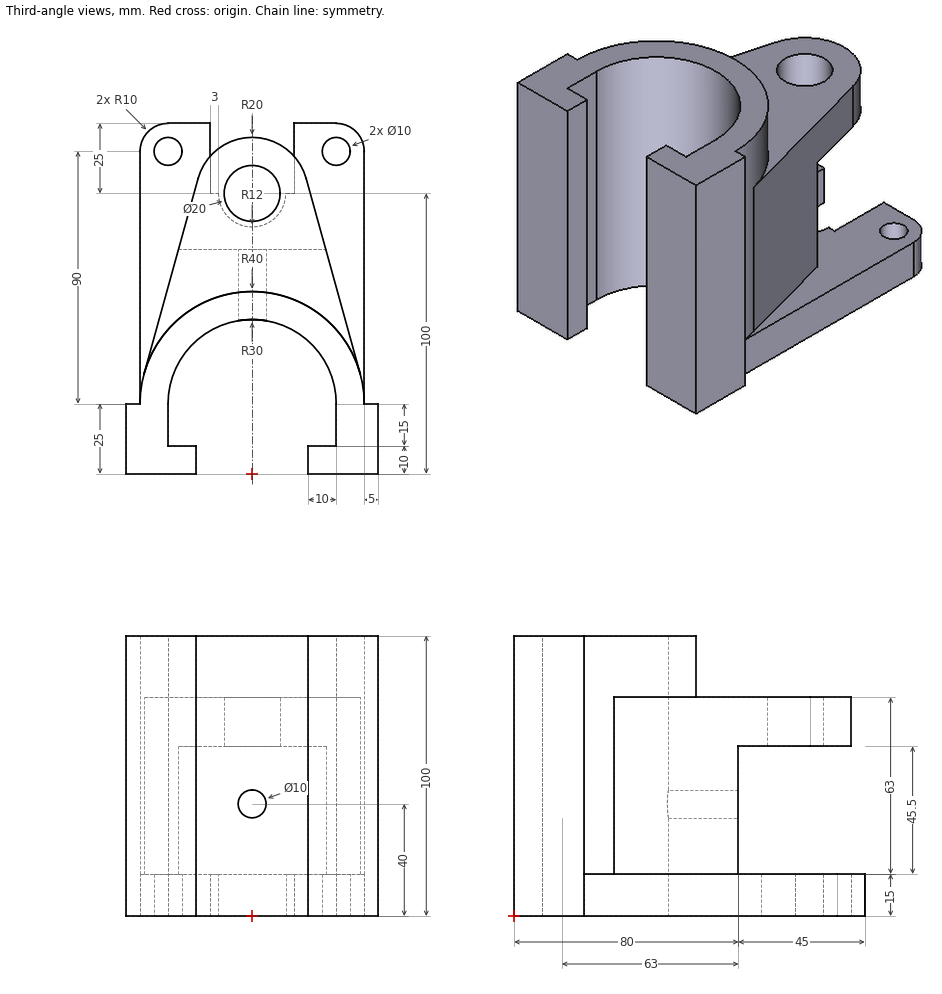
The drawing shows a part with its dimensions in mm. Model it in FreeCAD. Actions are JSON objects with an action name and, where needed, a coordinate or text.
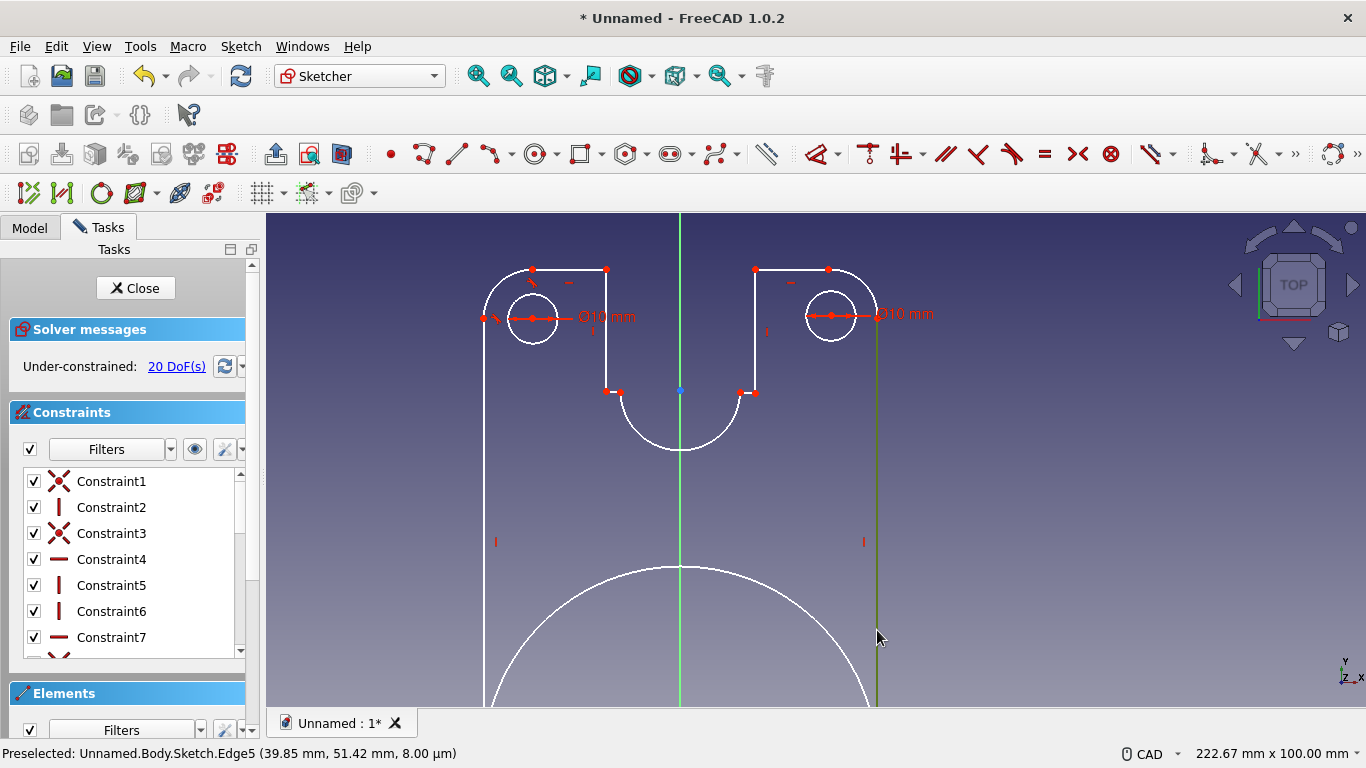
{"action": "left_click", "coordinate": [873, 296]}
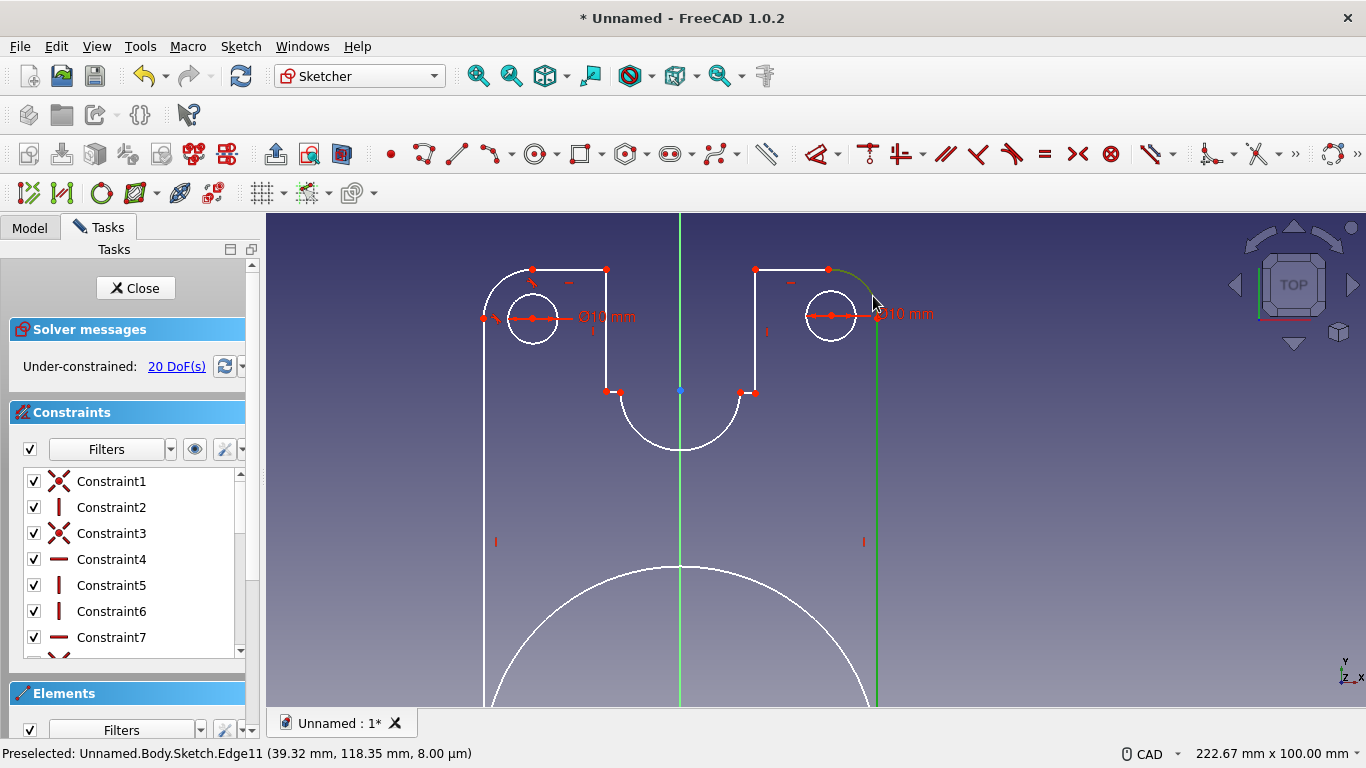
{"action": "key", "text": "t"}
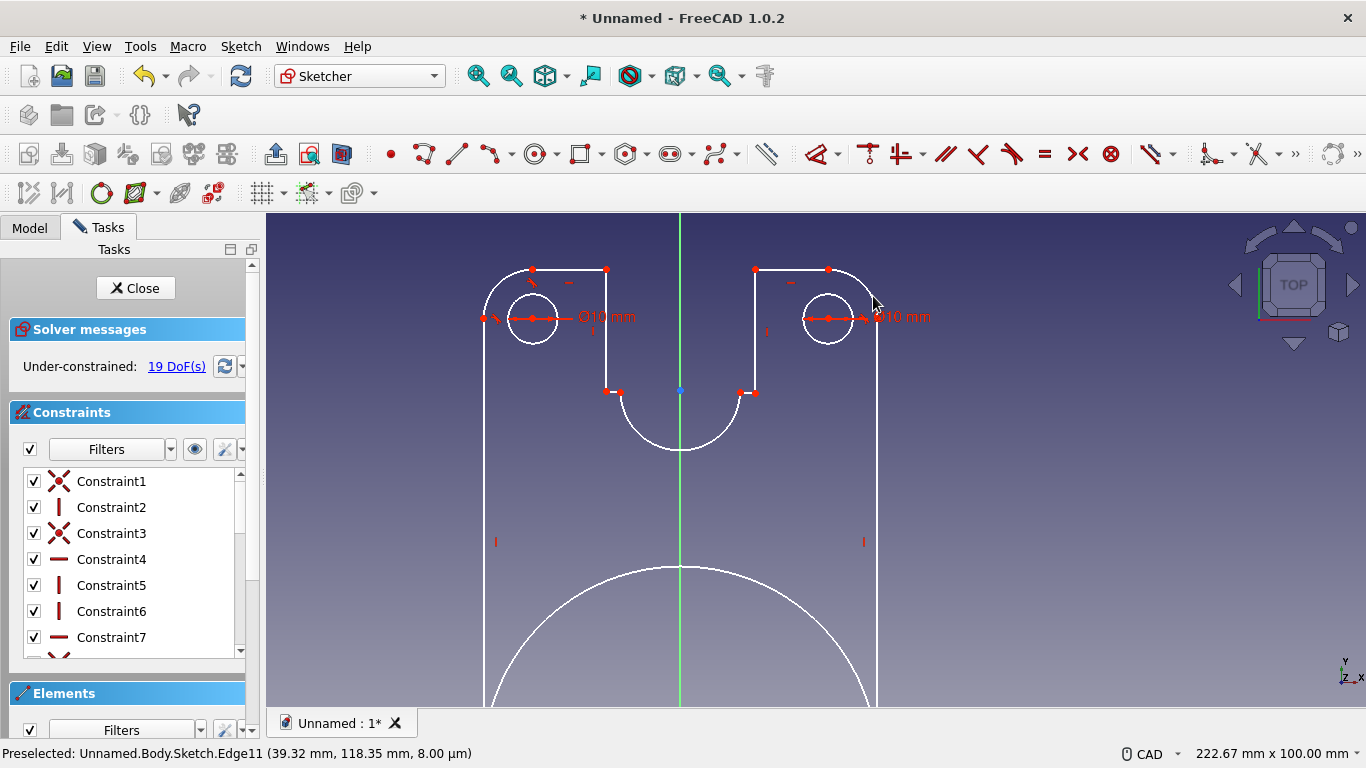
{"action": "left_click", "coordinate": [806, 270]}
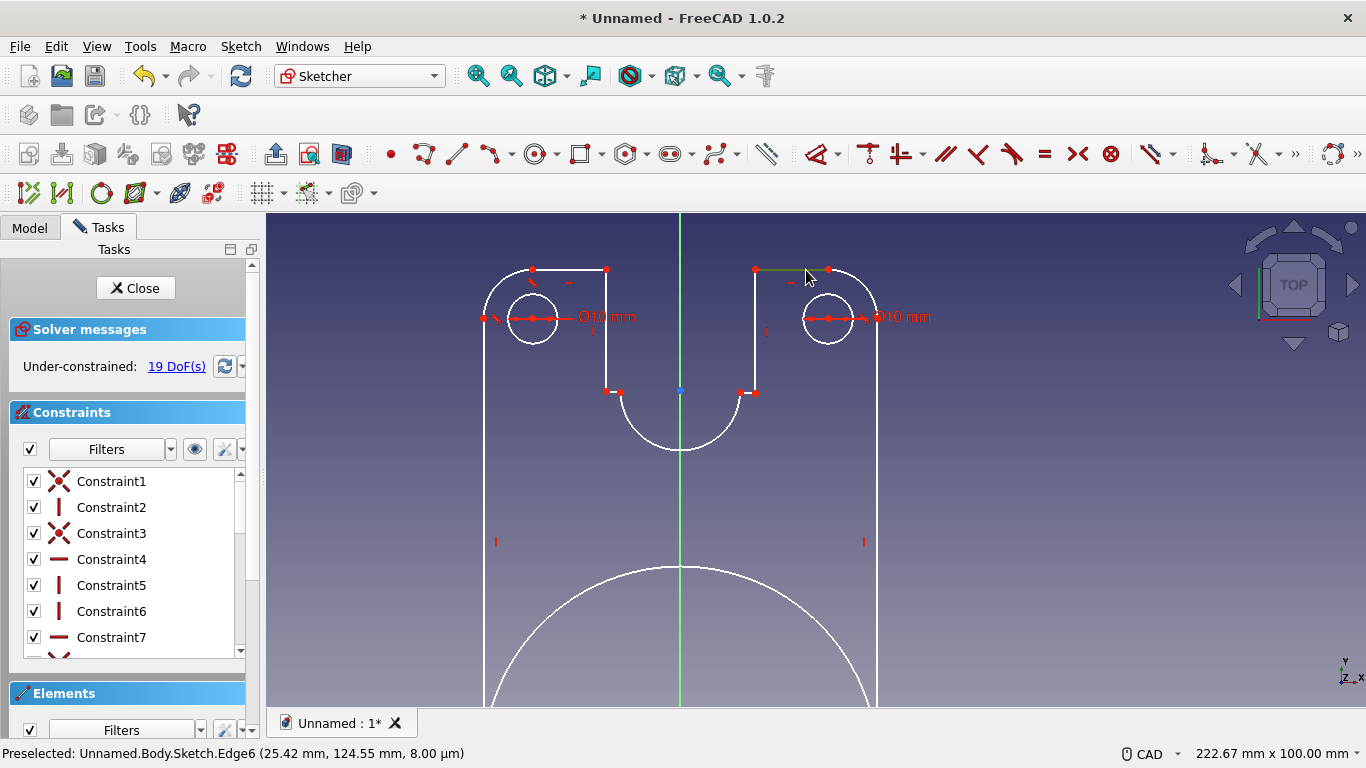
{"action": "left_click", "coordinate": [872, 297]}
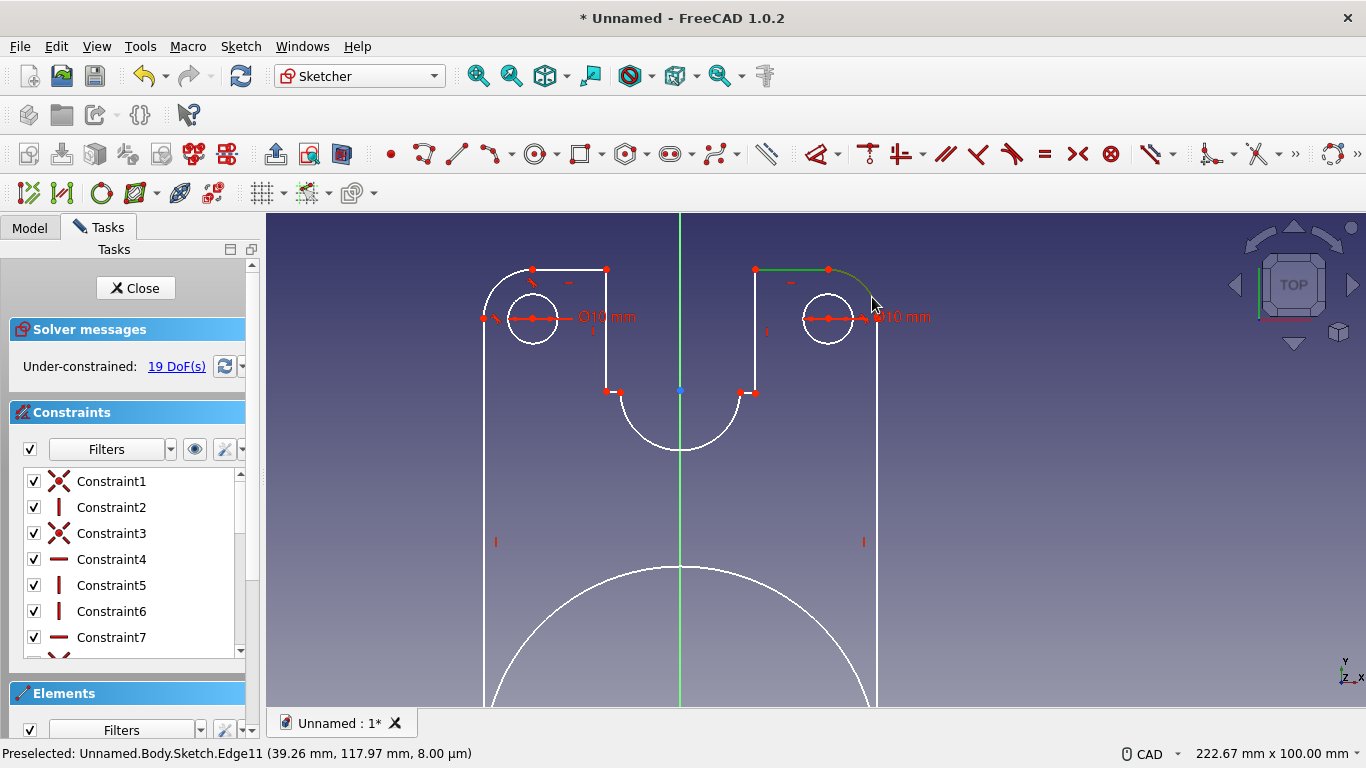
{"action": "key", "text": "t"}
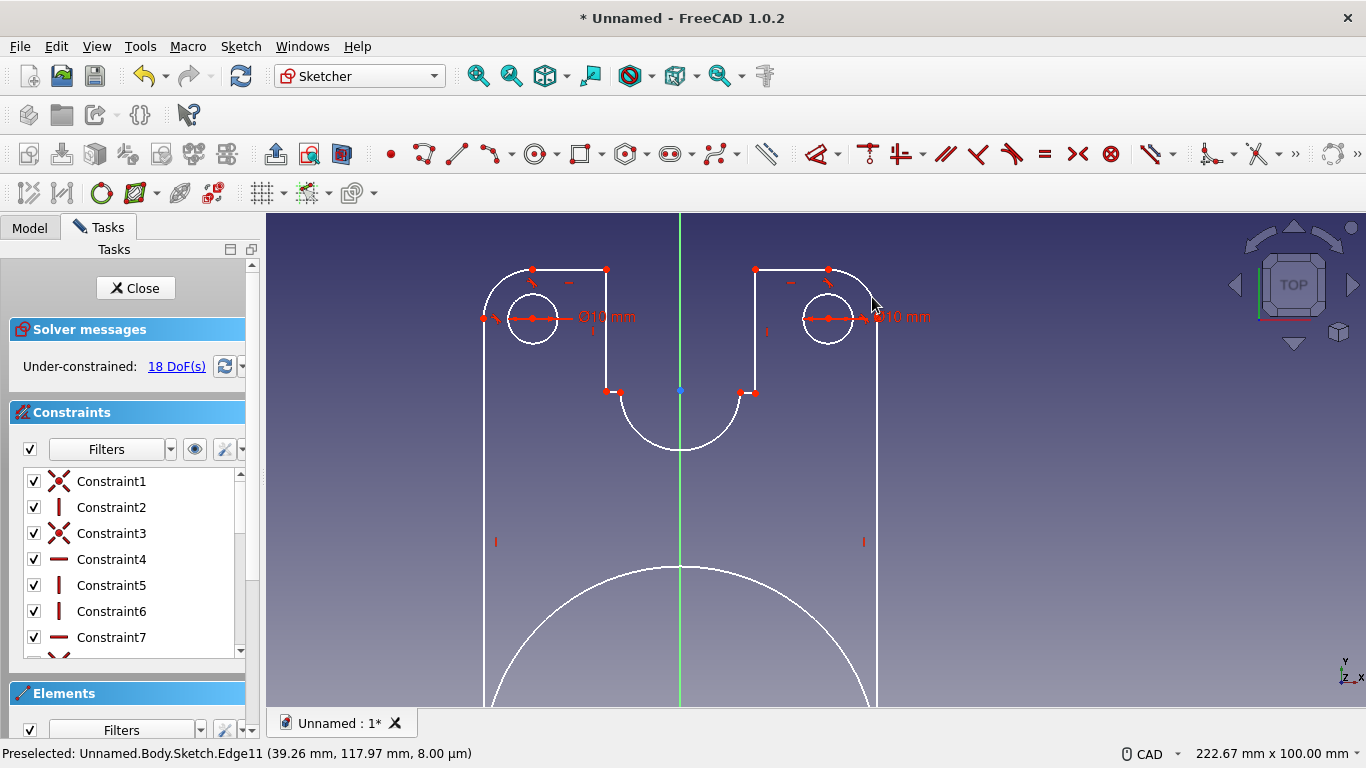
{"action": "scroll", "coordinate": [613, 392], "scroll_direction": "up", "scroll_amount": 4}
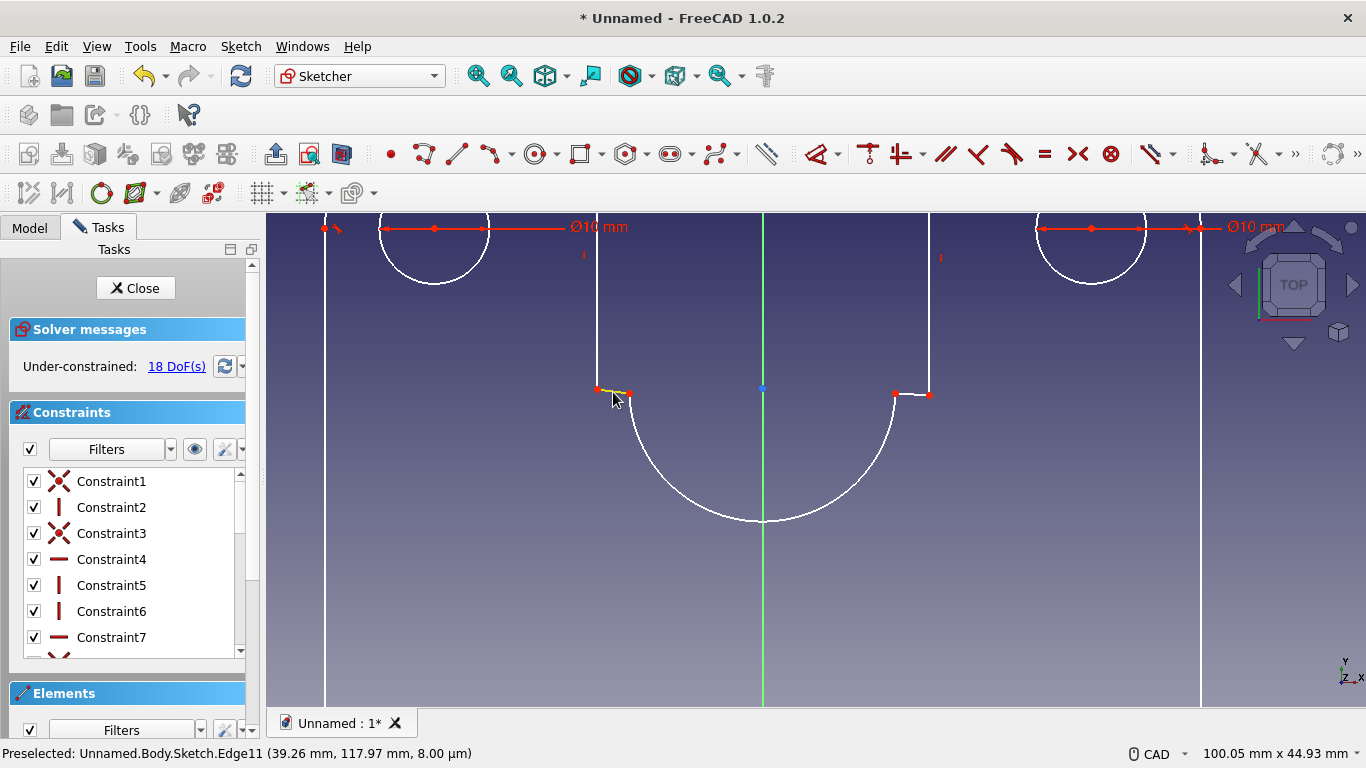
{"action": "left_click", "coordinate": [613, 392]}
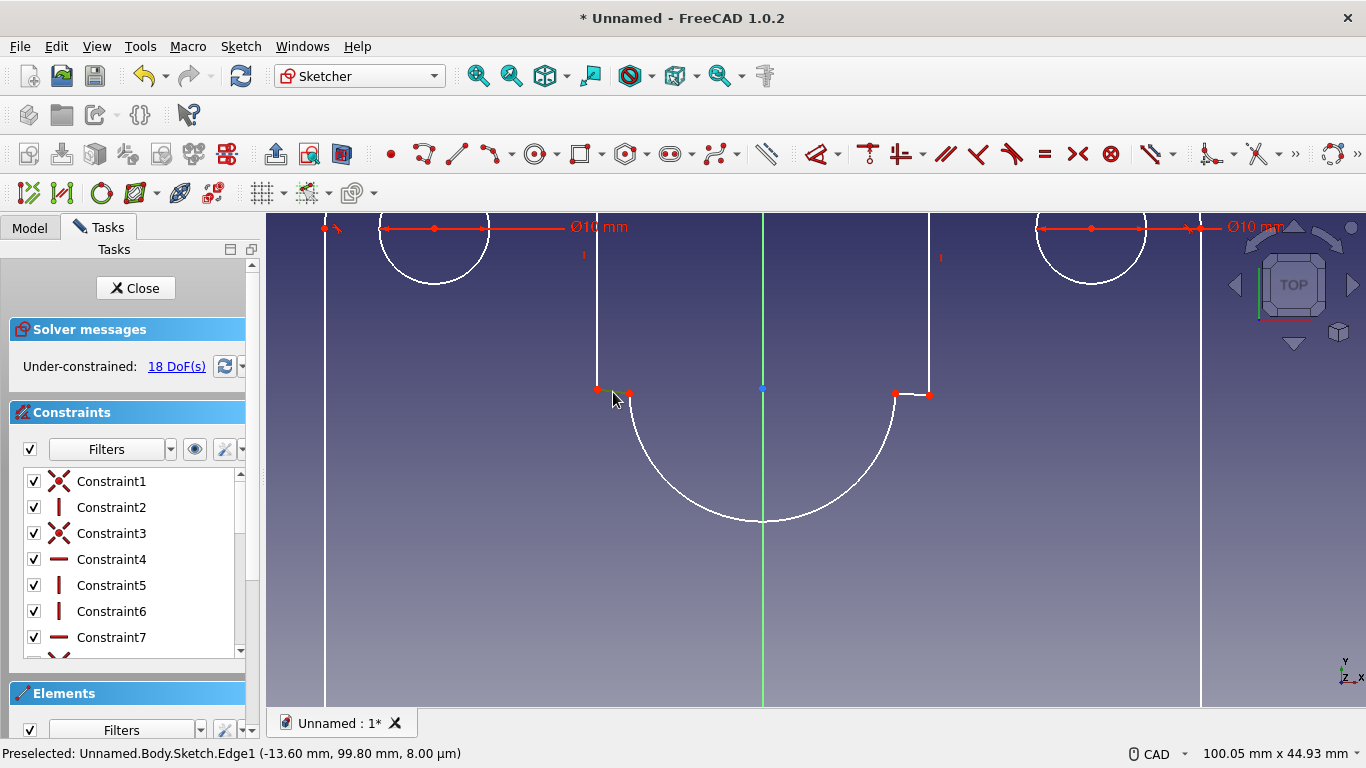
{"action": "key", "text": "h"}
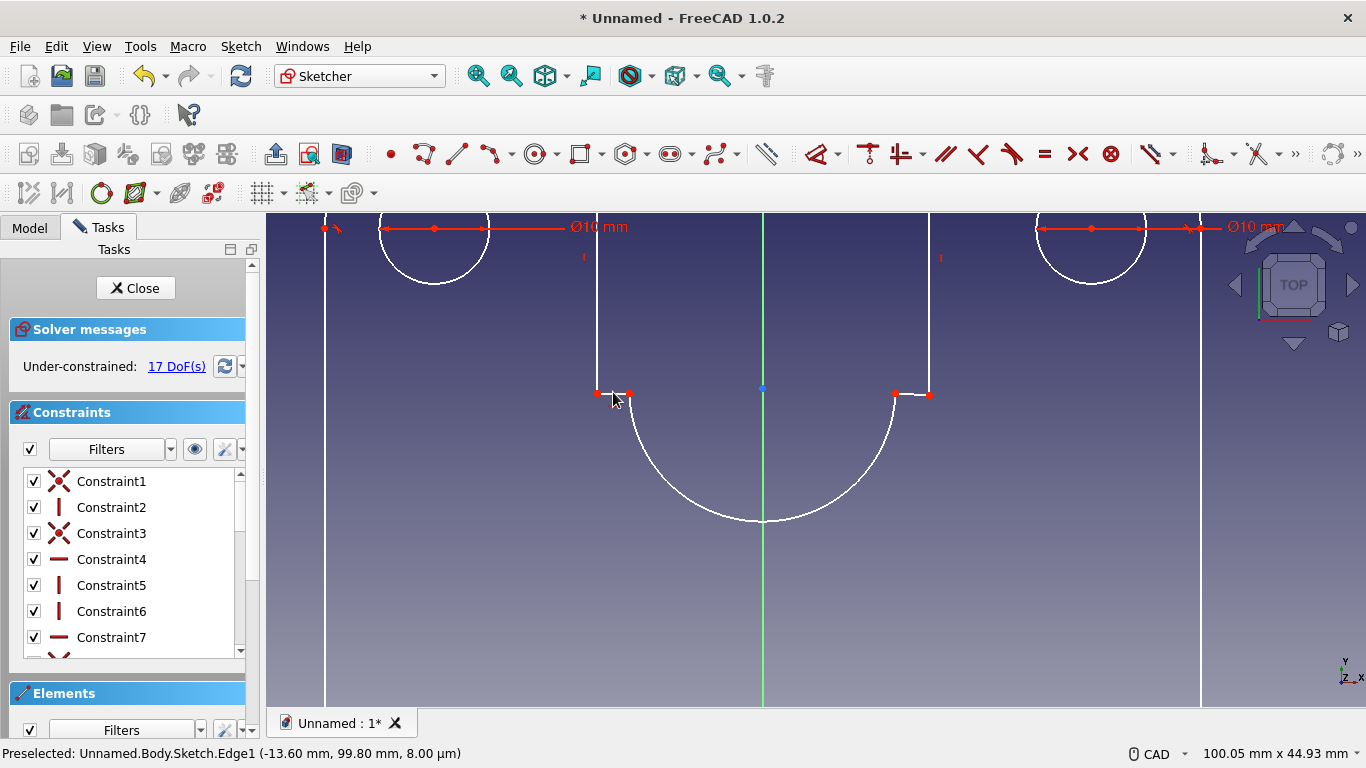
{"action": "scroll", "coordinate": [919, 395], "scroll_direction": "up", "scroll_amount": 2}